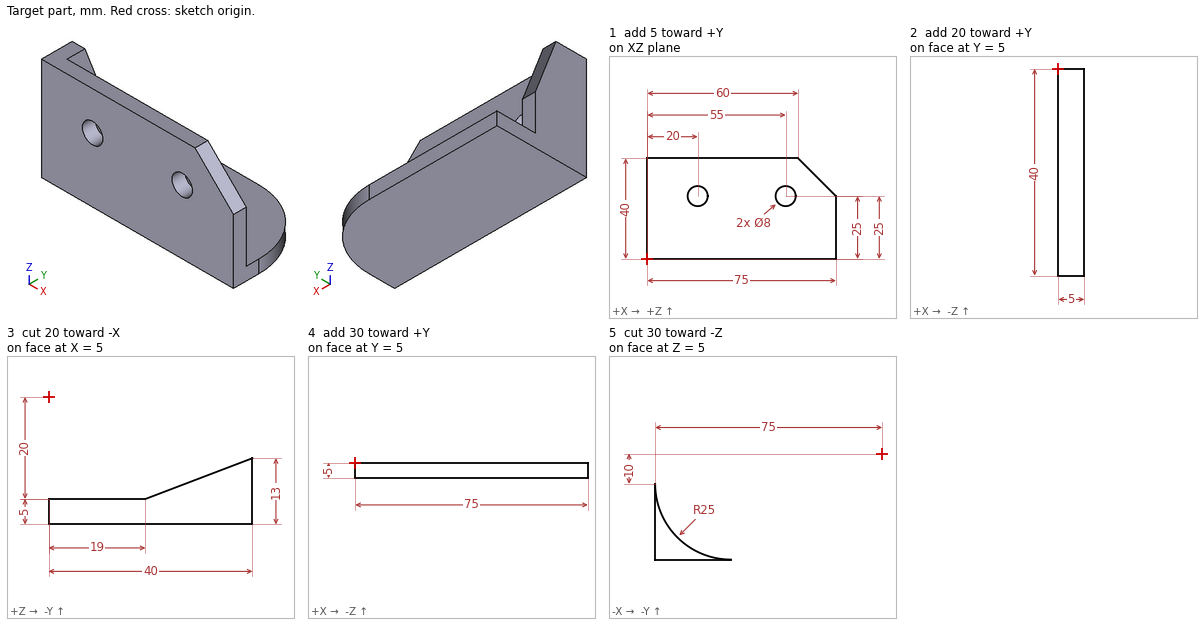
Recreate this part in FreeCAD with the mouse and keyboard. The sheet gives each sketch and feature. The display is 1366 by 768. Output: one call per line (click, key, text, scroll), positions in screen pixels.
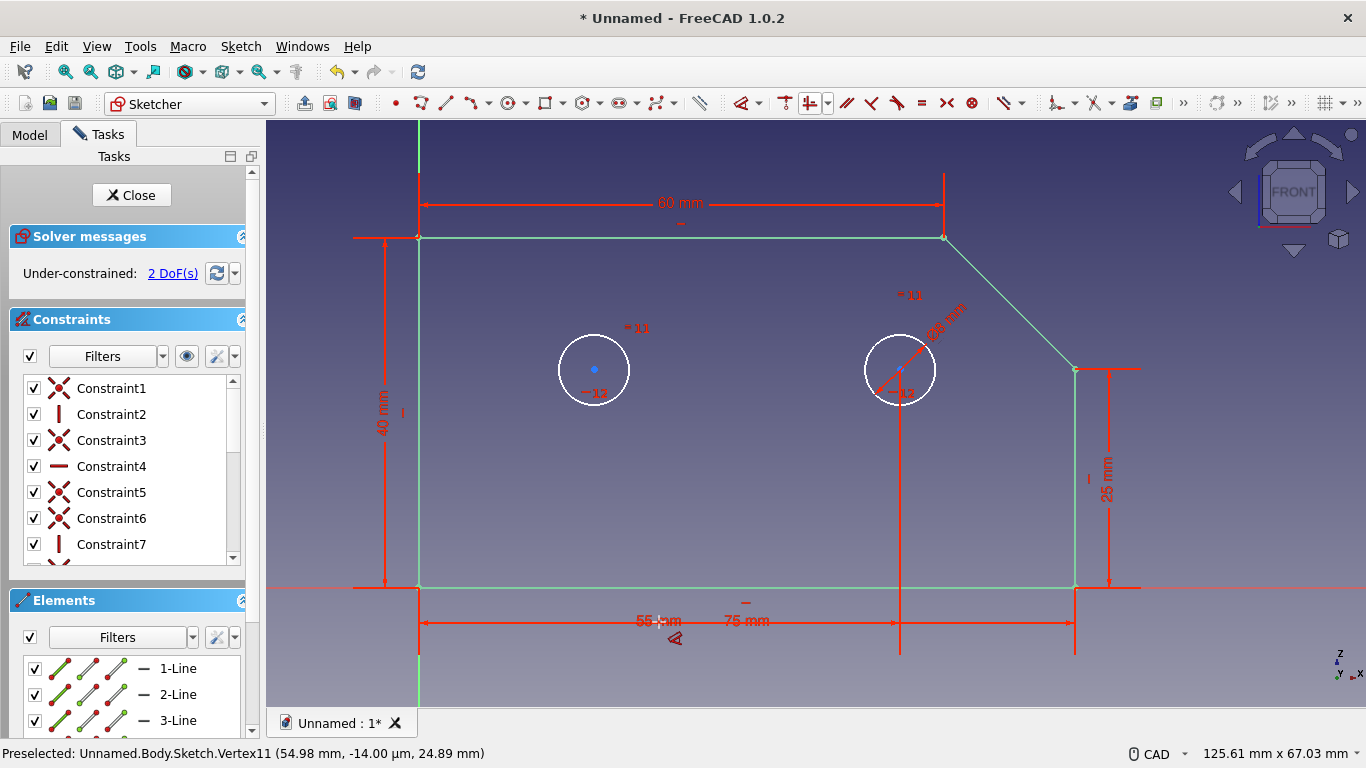
click(900, 370)
click(385, 479)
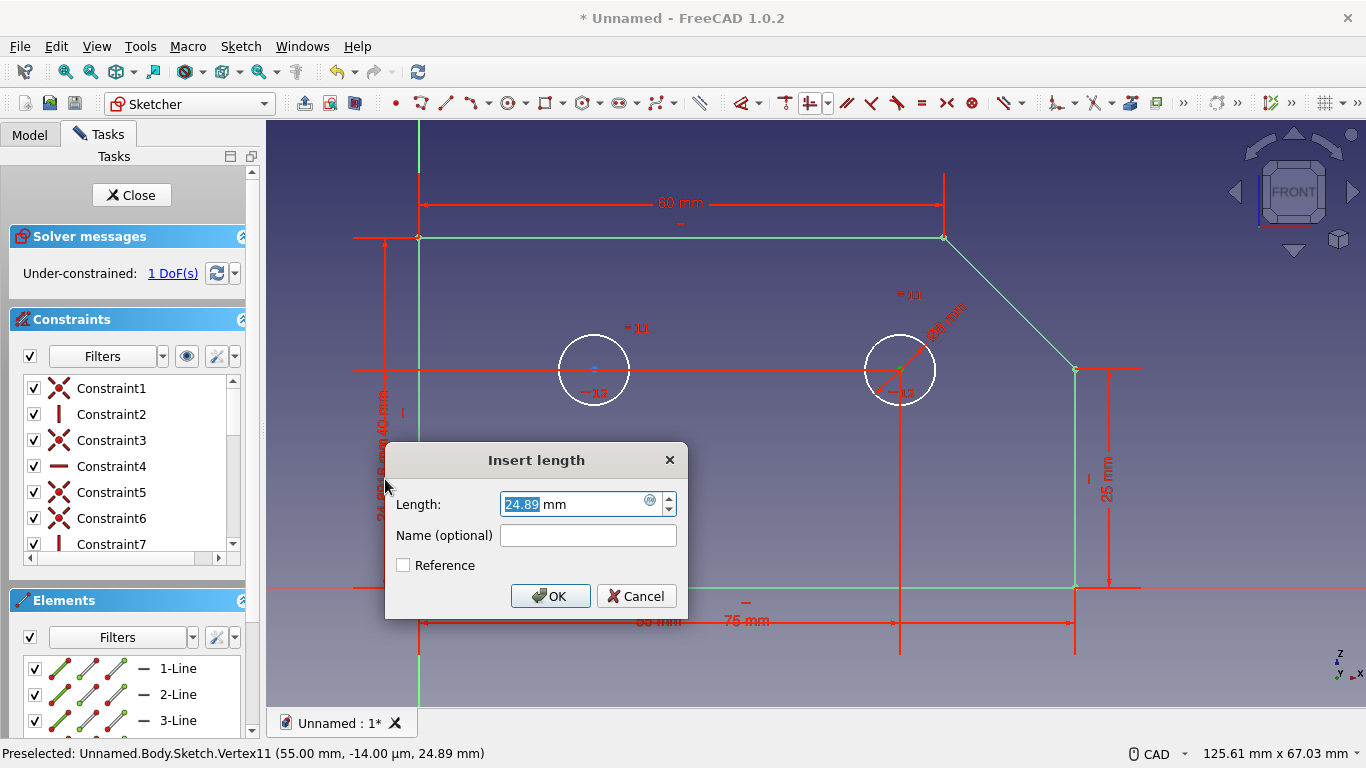
text(25)
key(Return)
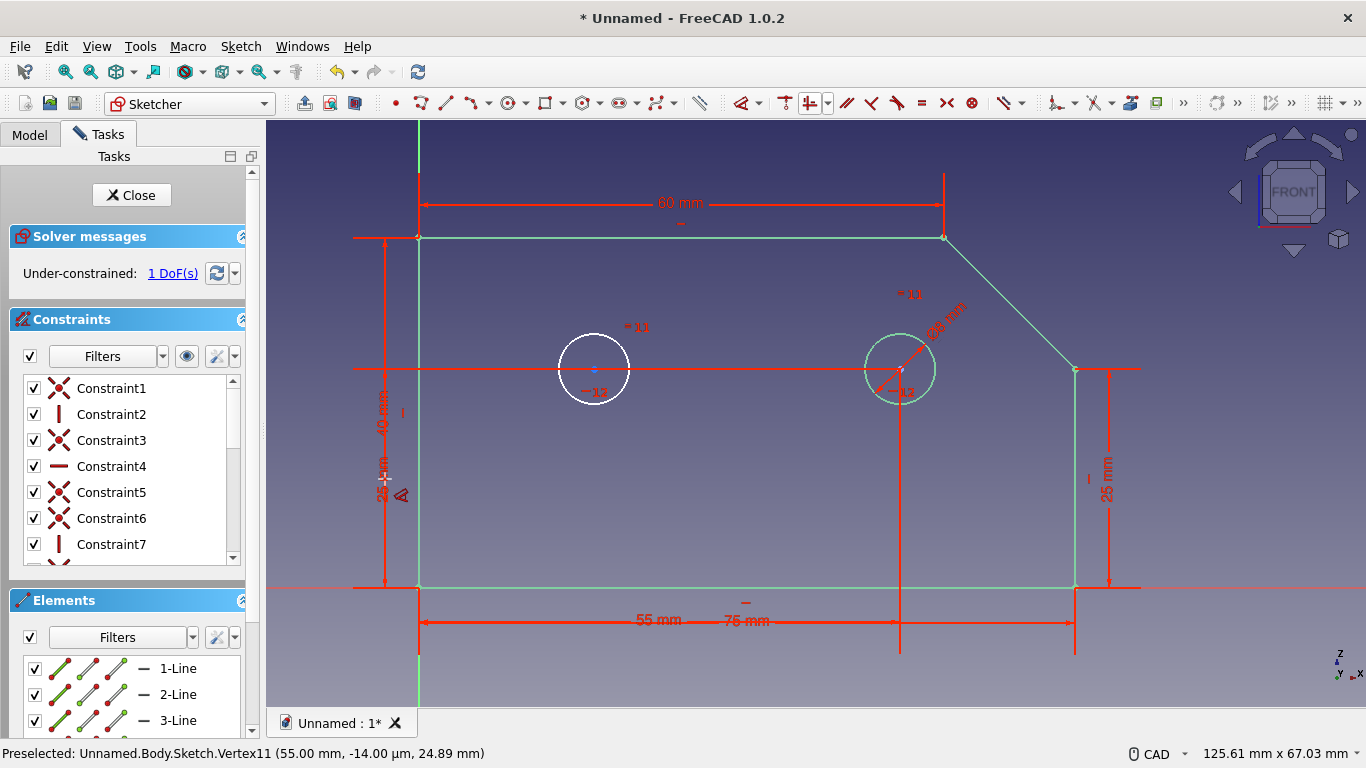
click(594, 369)
click(506, 622)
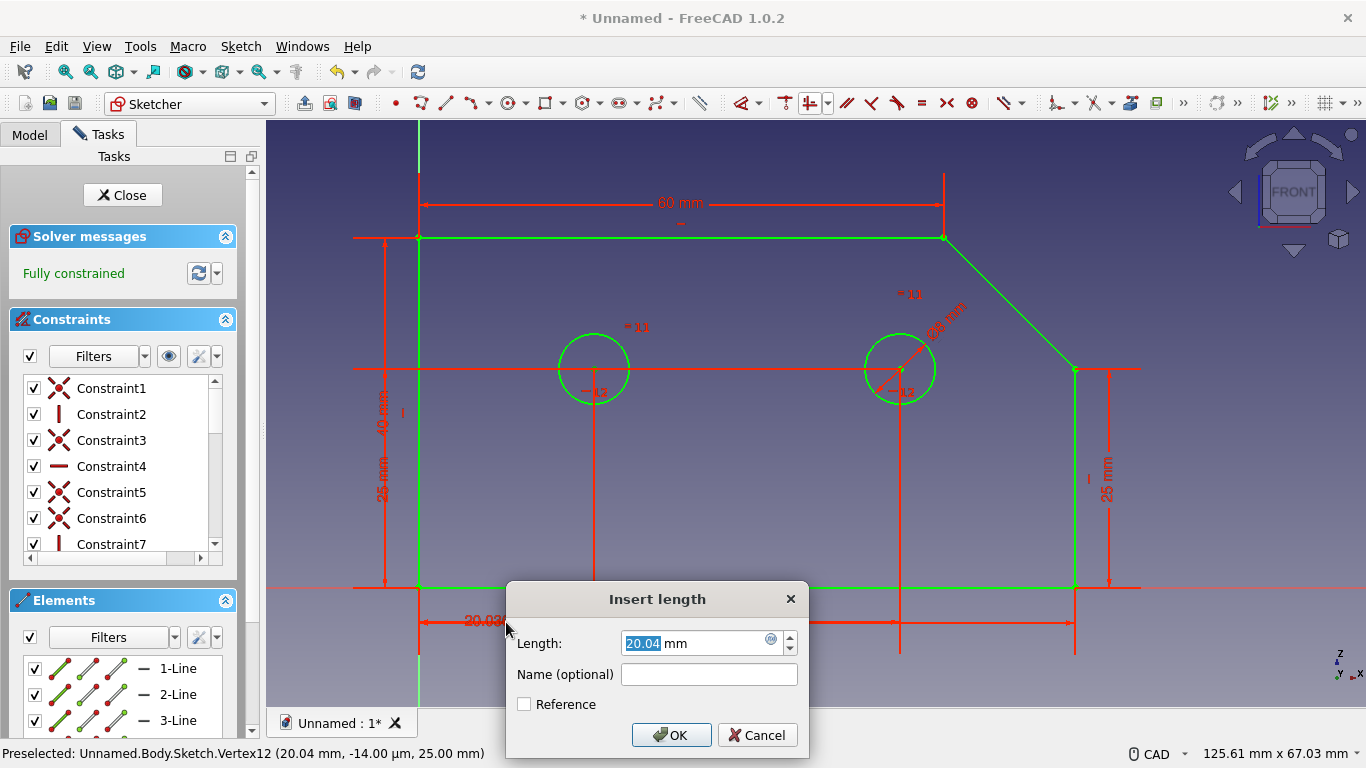
text(20)
key(Return)
key(Escape)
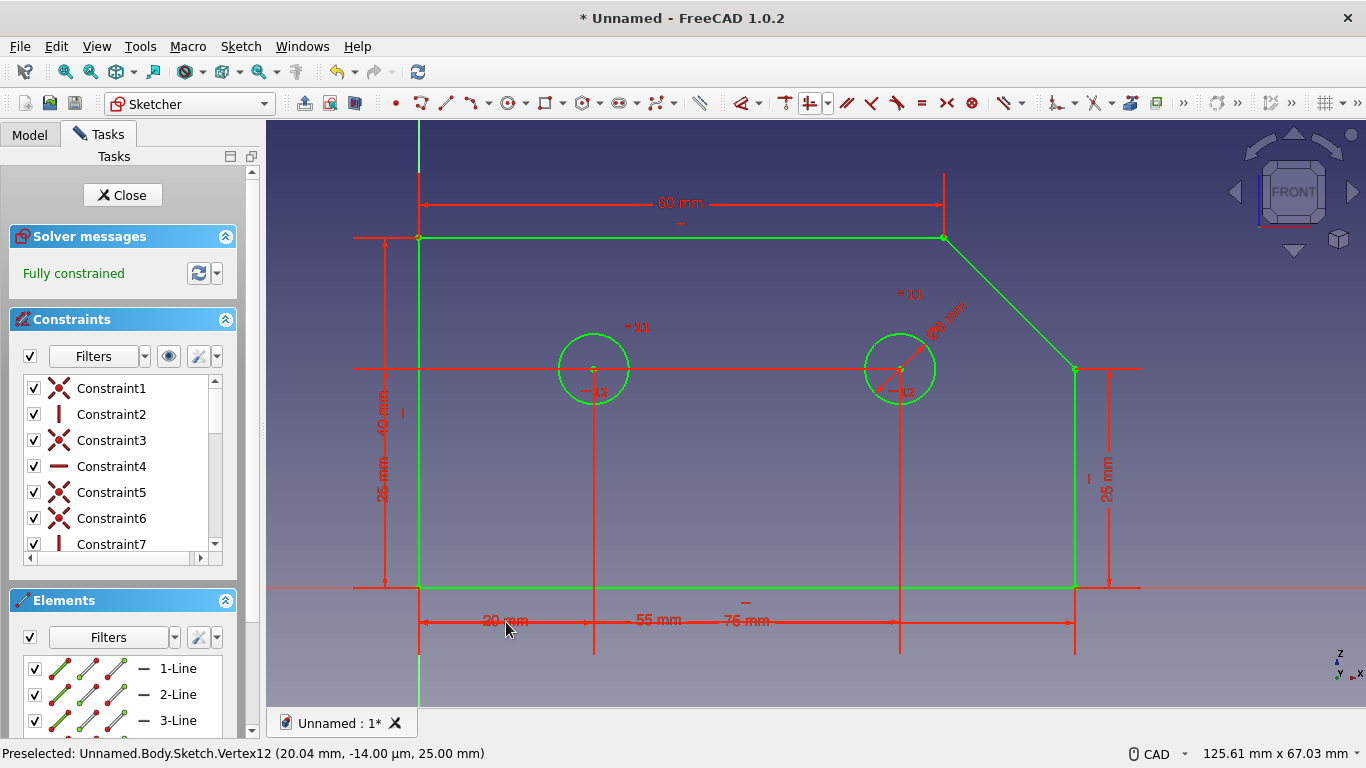
click(123, 195)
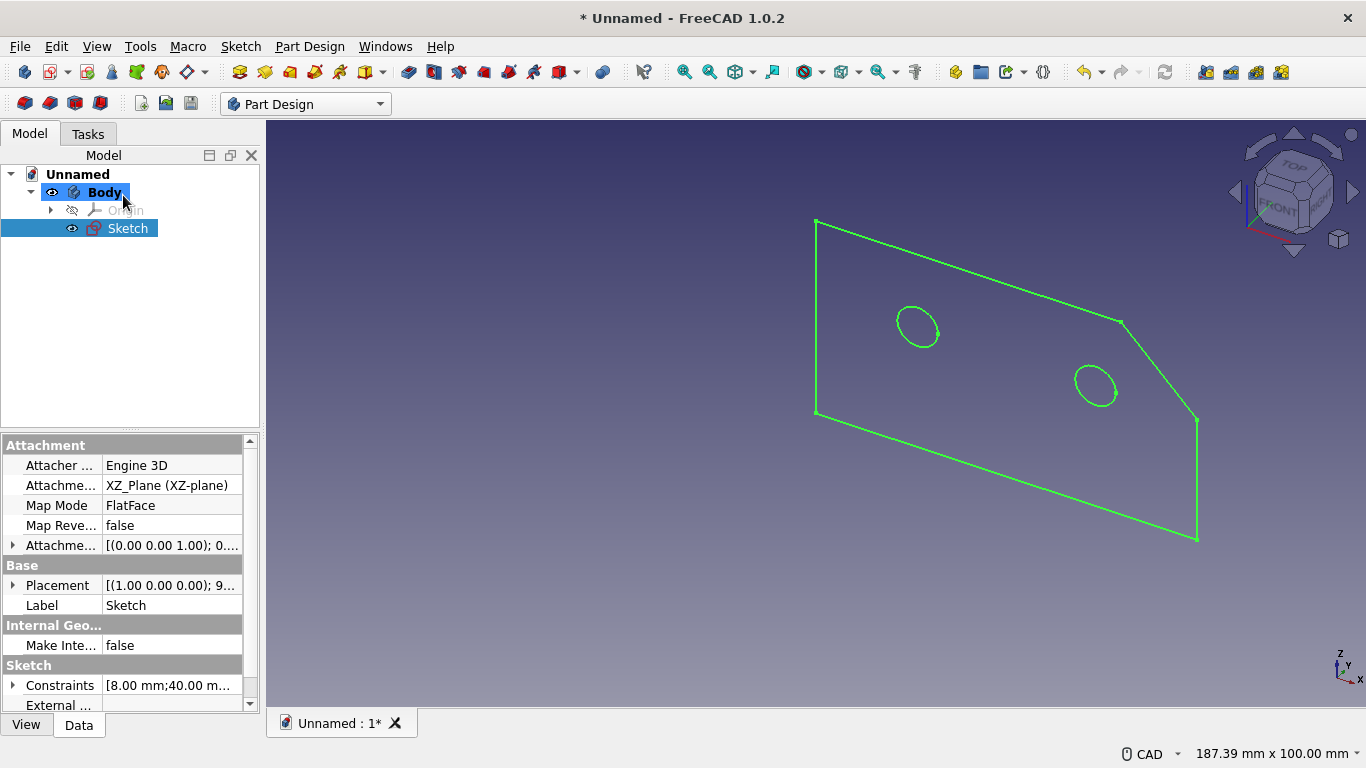
click(240, 72)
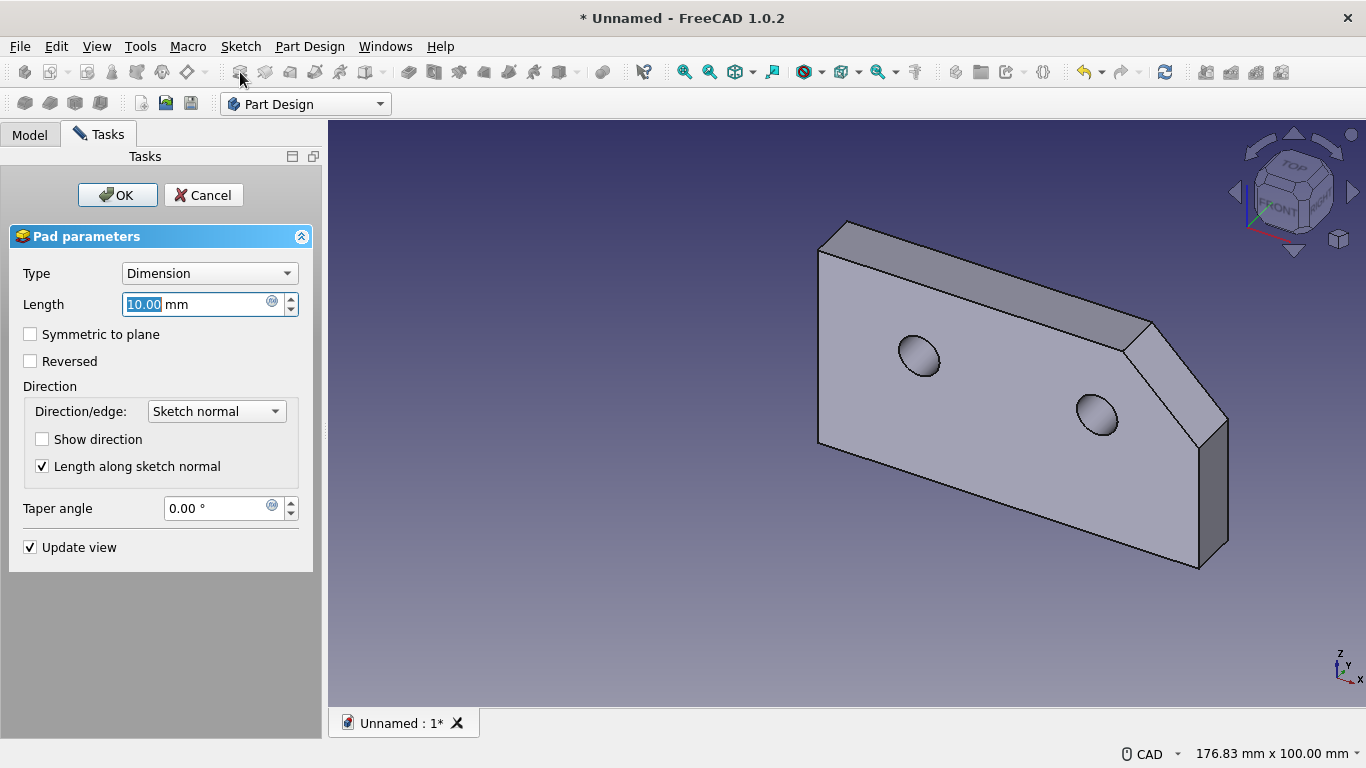
text(5)
key(Tab)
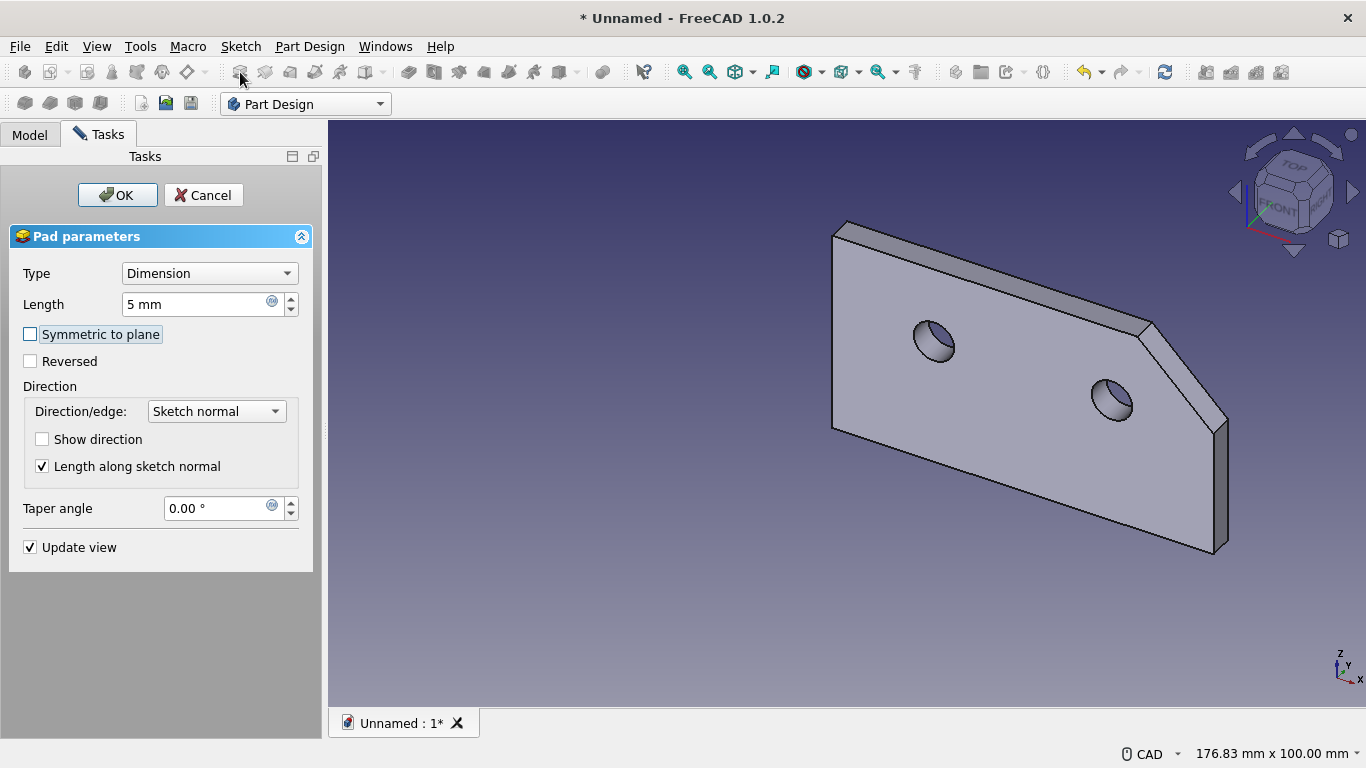
click(31, 361)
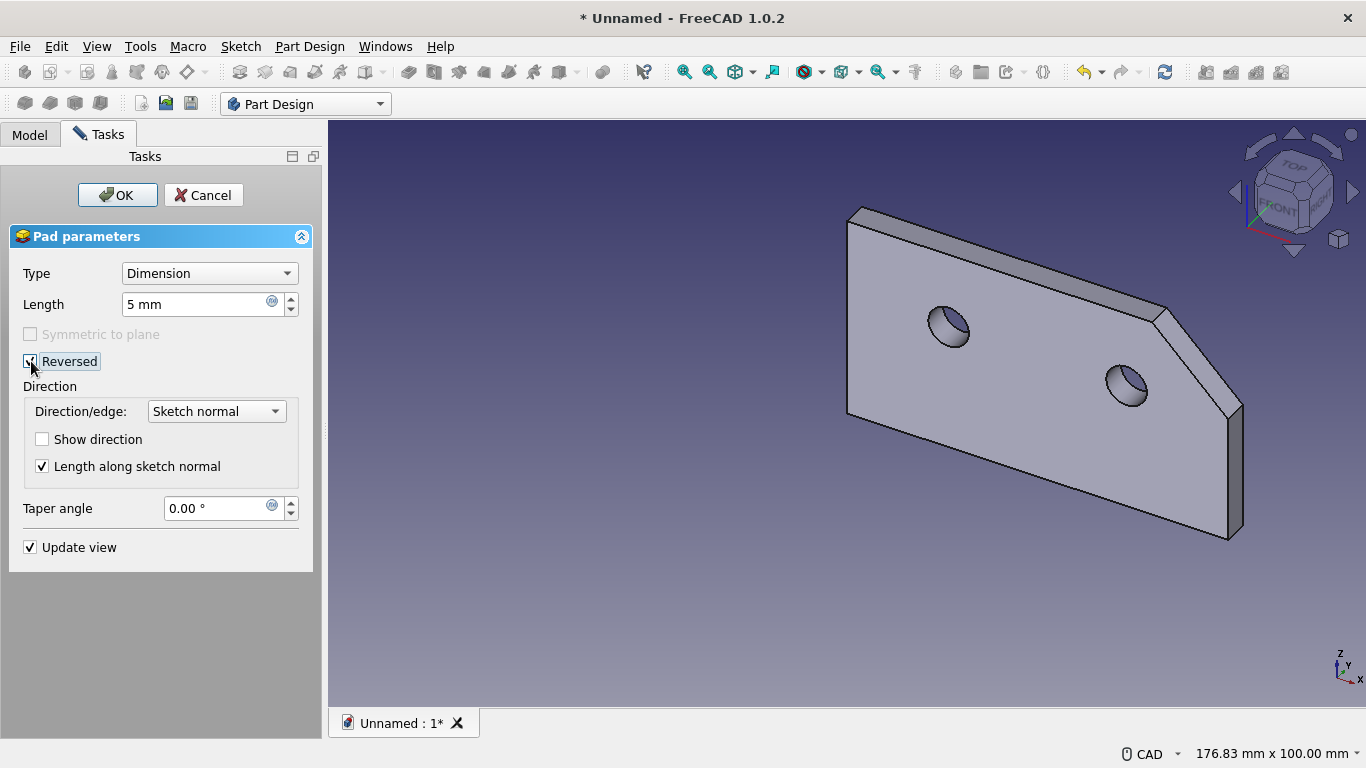
click(118, 195)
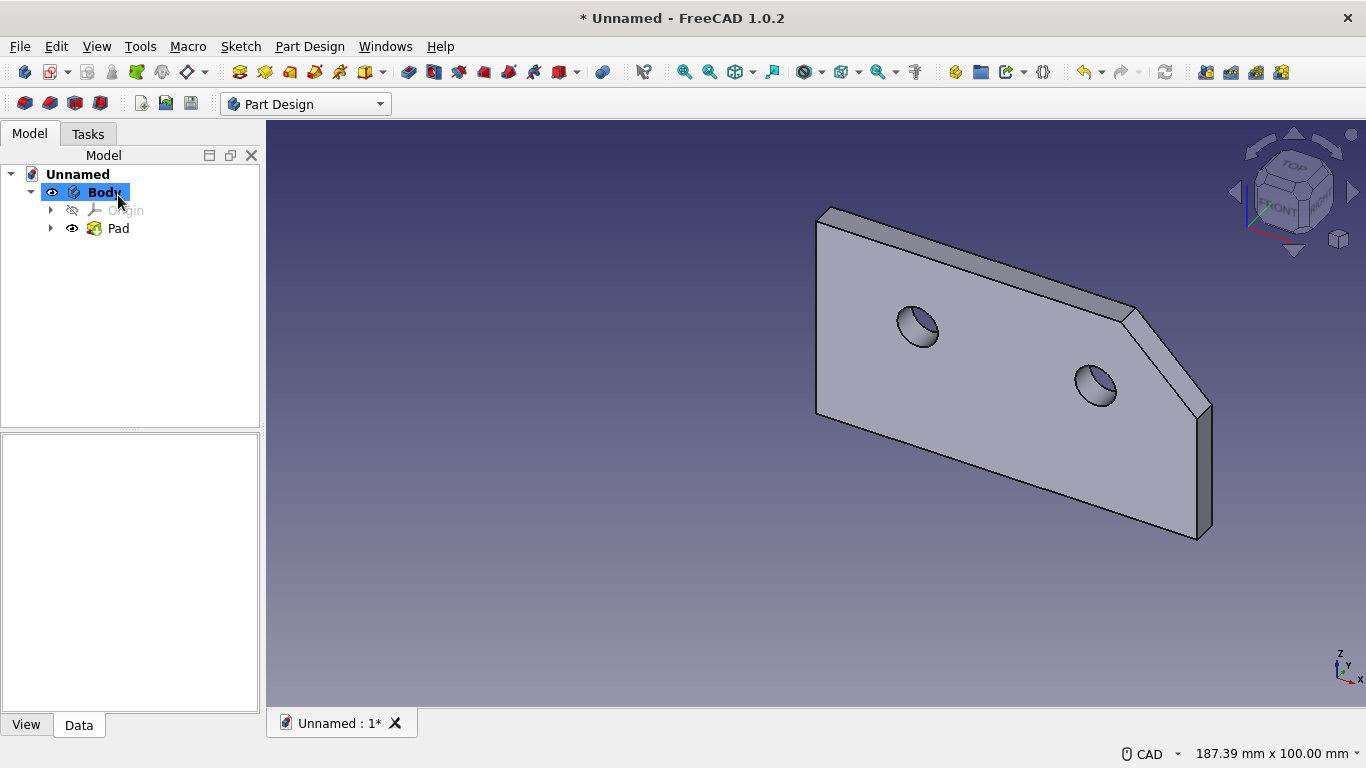
key(4)